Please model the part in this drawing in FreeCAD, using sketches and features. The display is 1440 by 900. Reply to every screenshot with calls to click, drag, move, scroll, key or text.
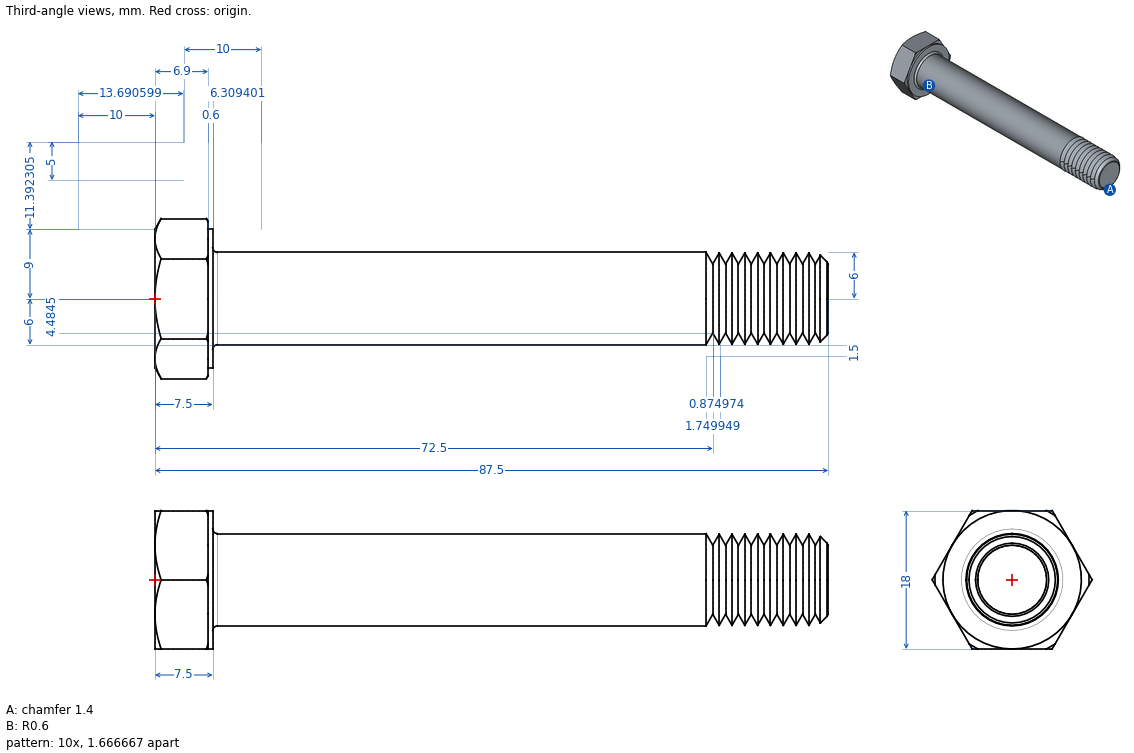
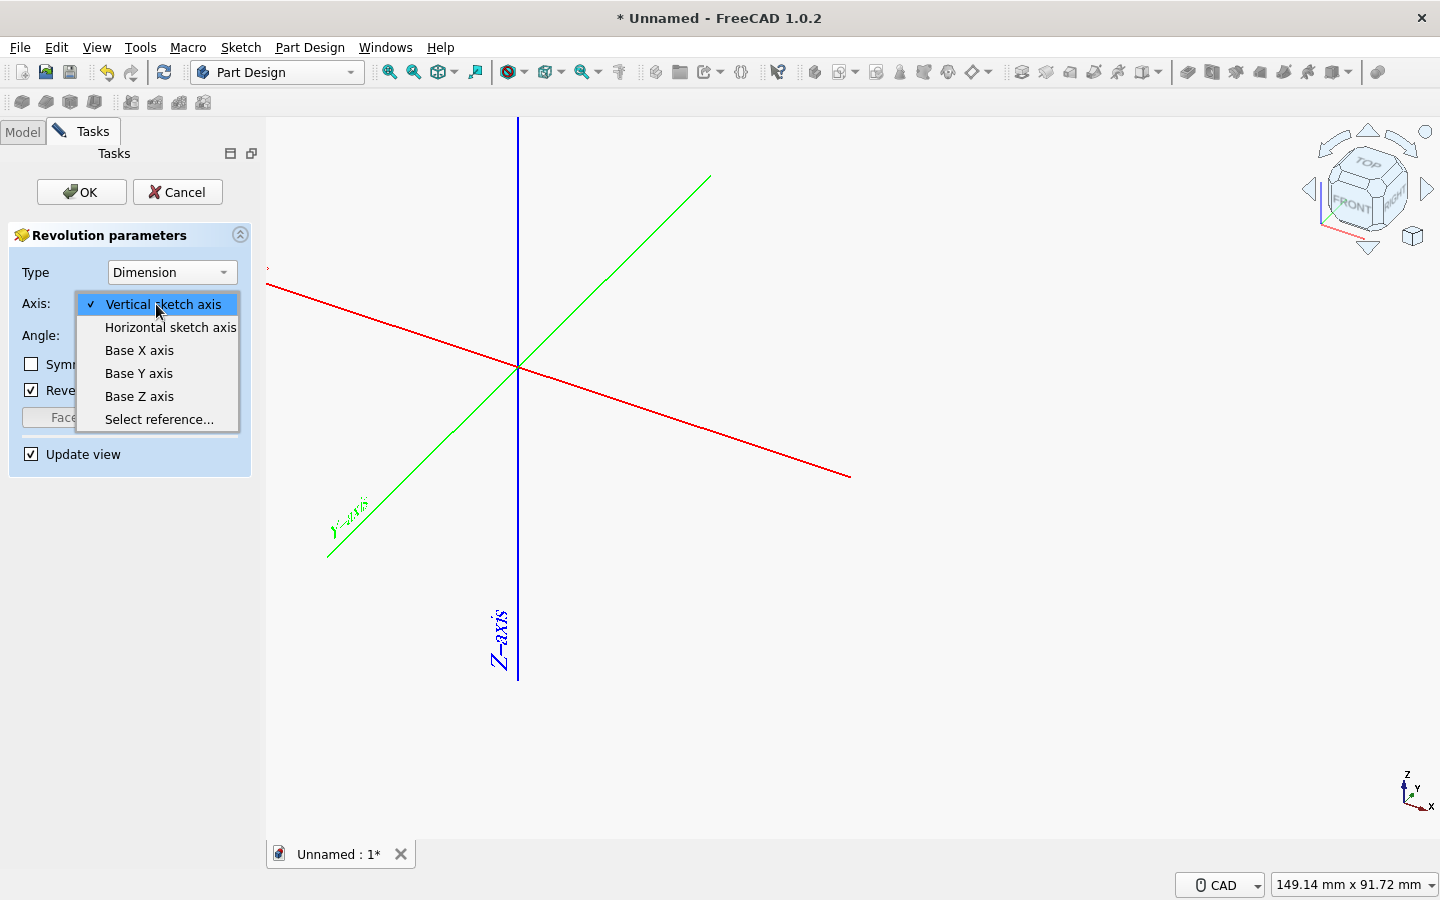
click(156, 328)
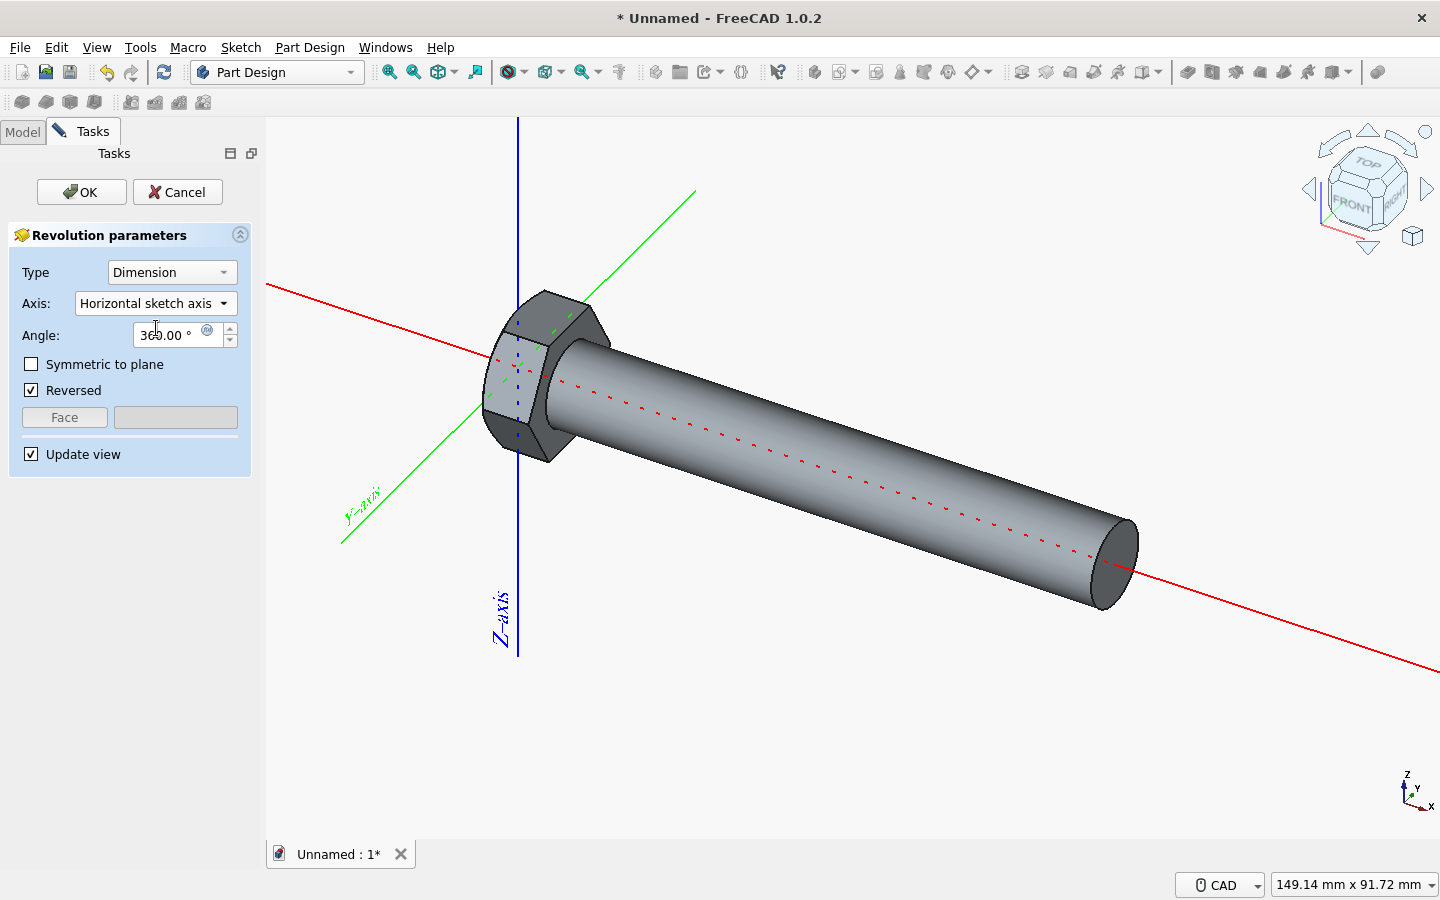
click(82, 192)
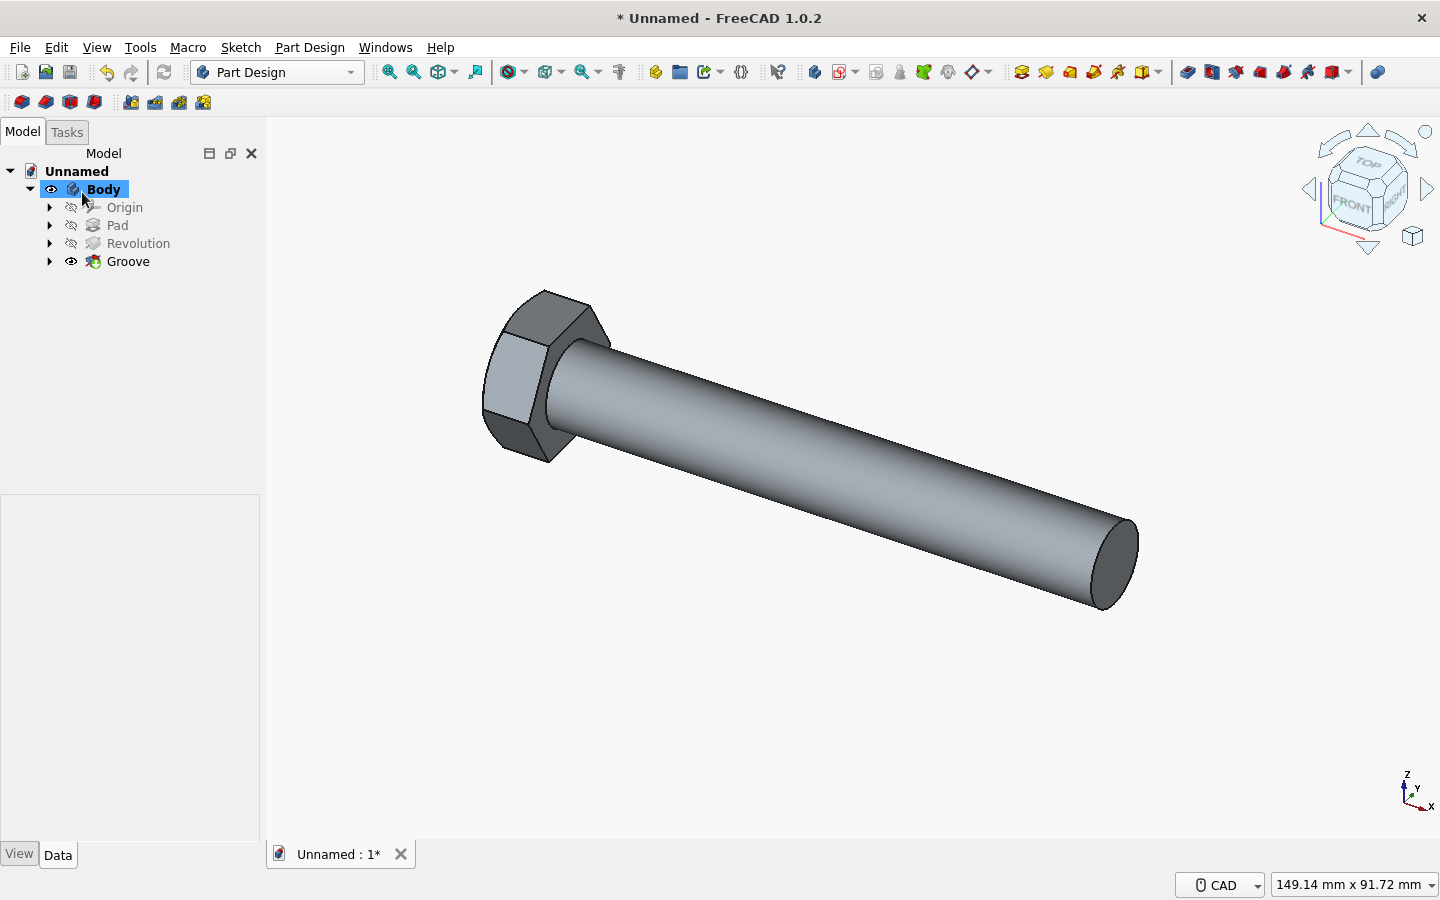
click(840, 72)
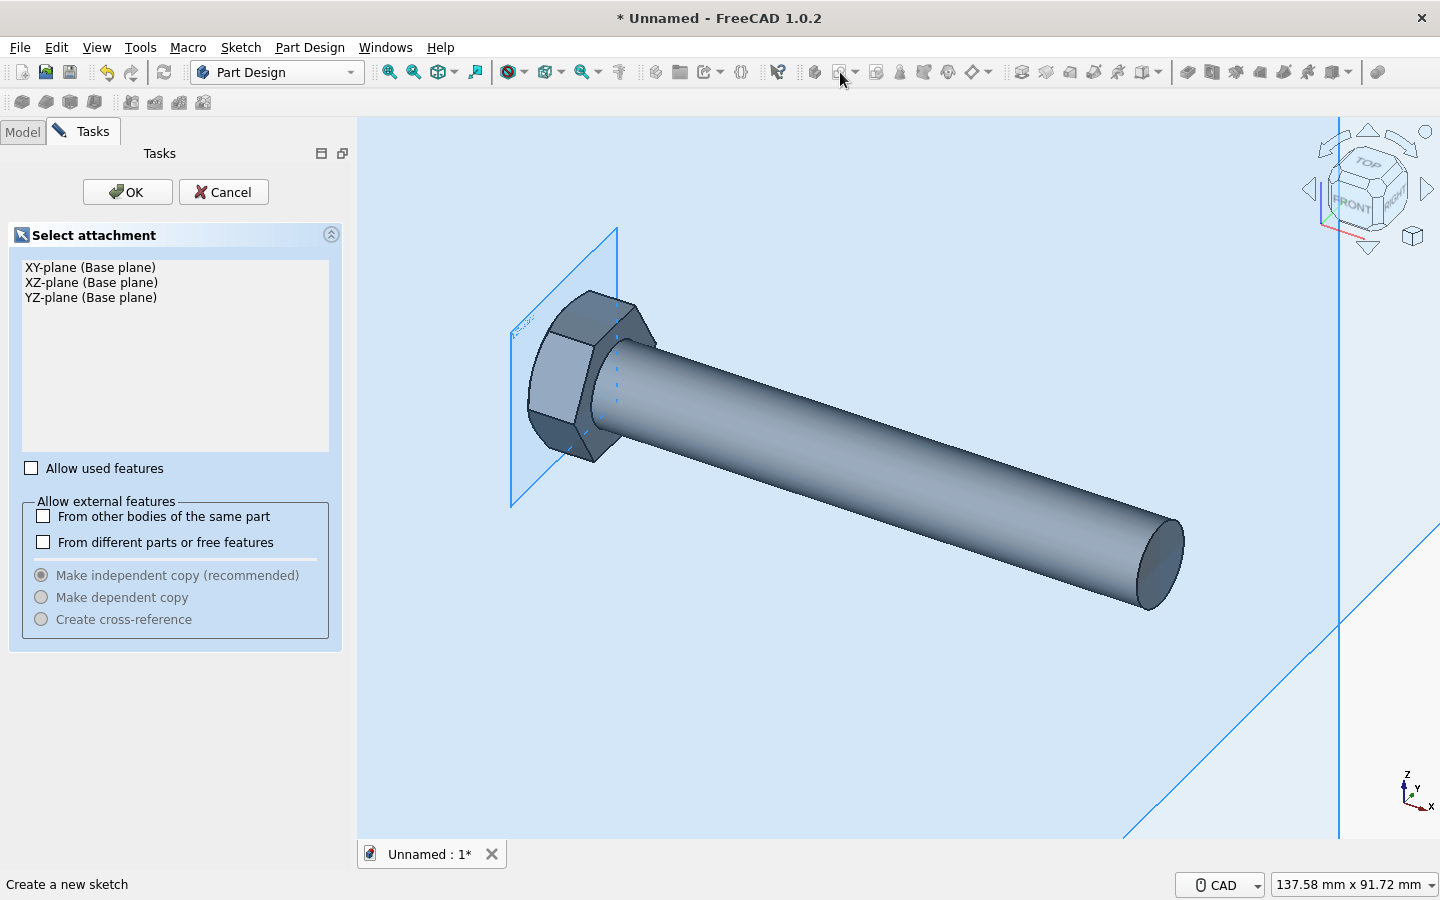
click(82, 268)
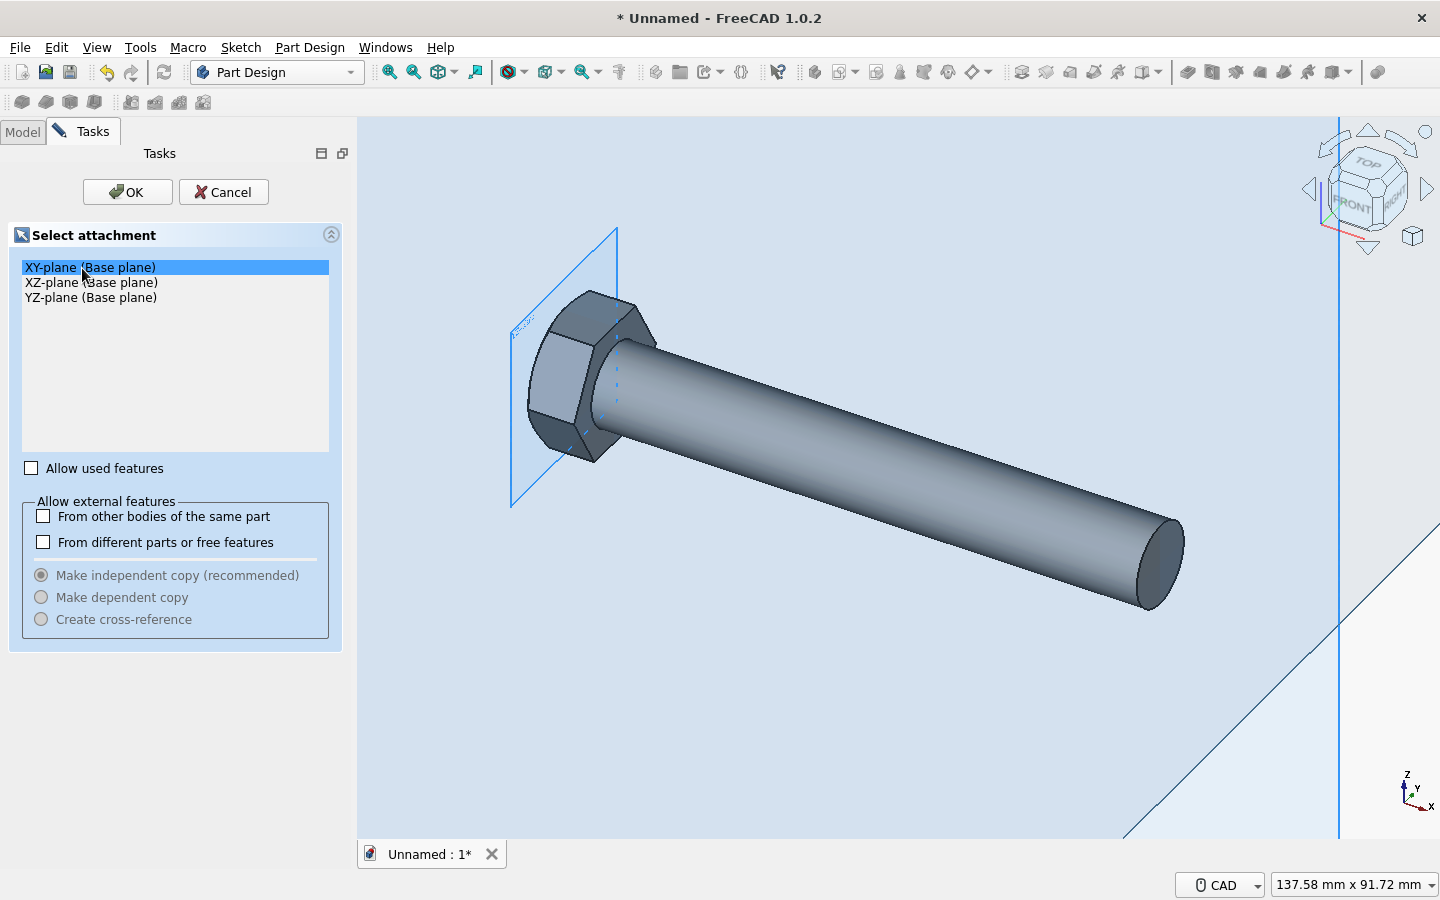
click(128, 192)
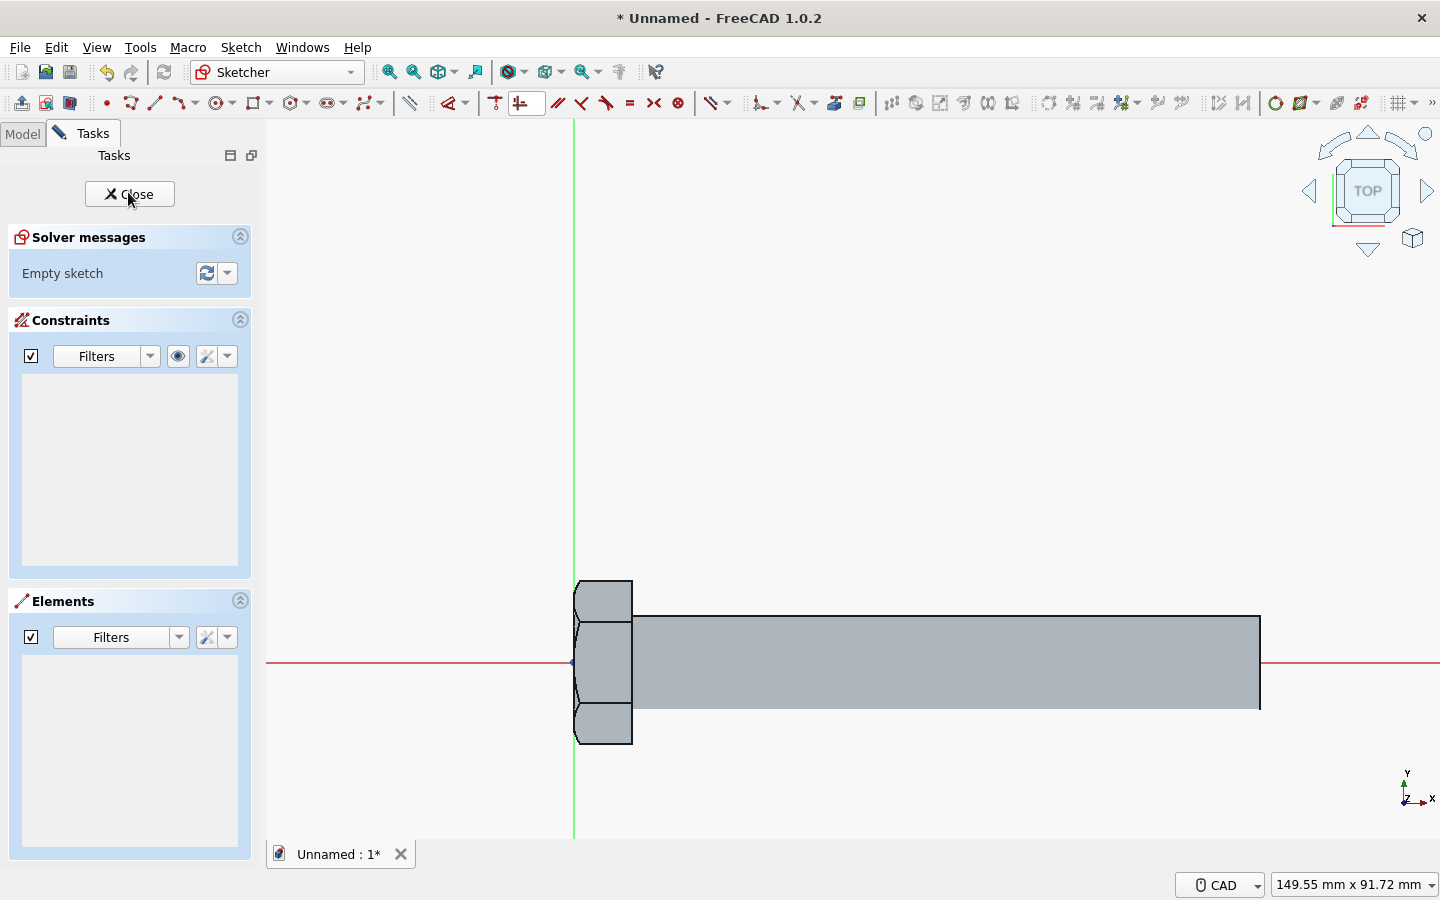
click(70, 104)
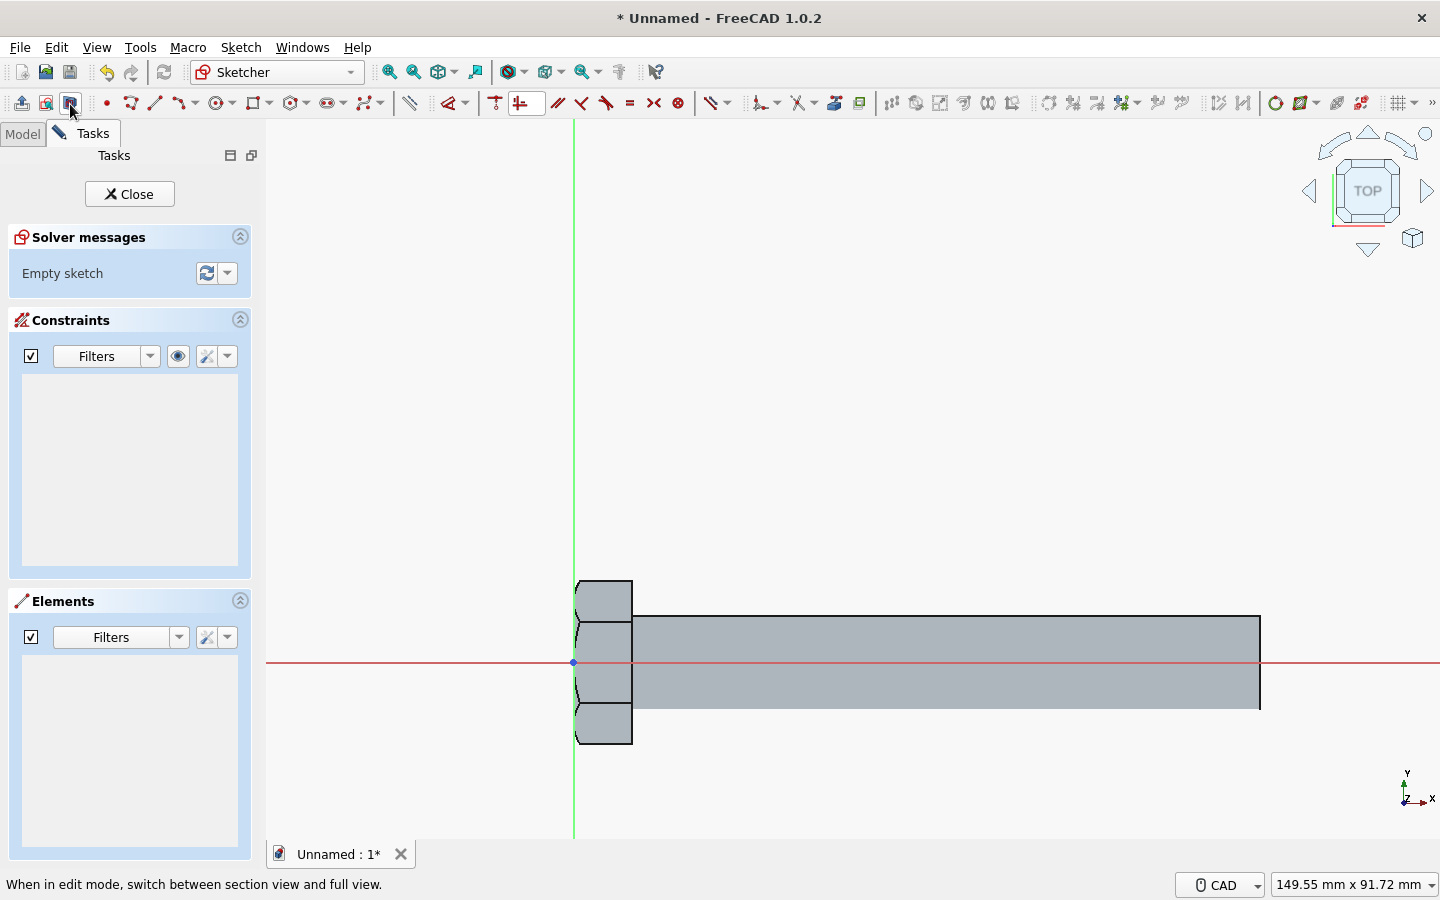
scroll(537, 643, up, 5)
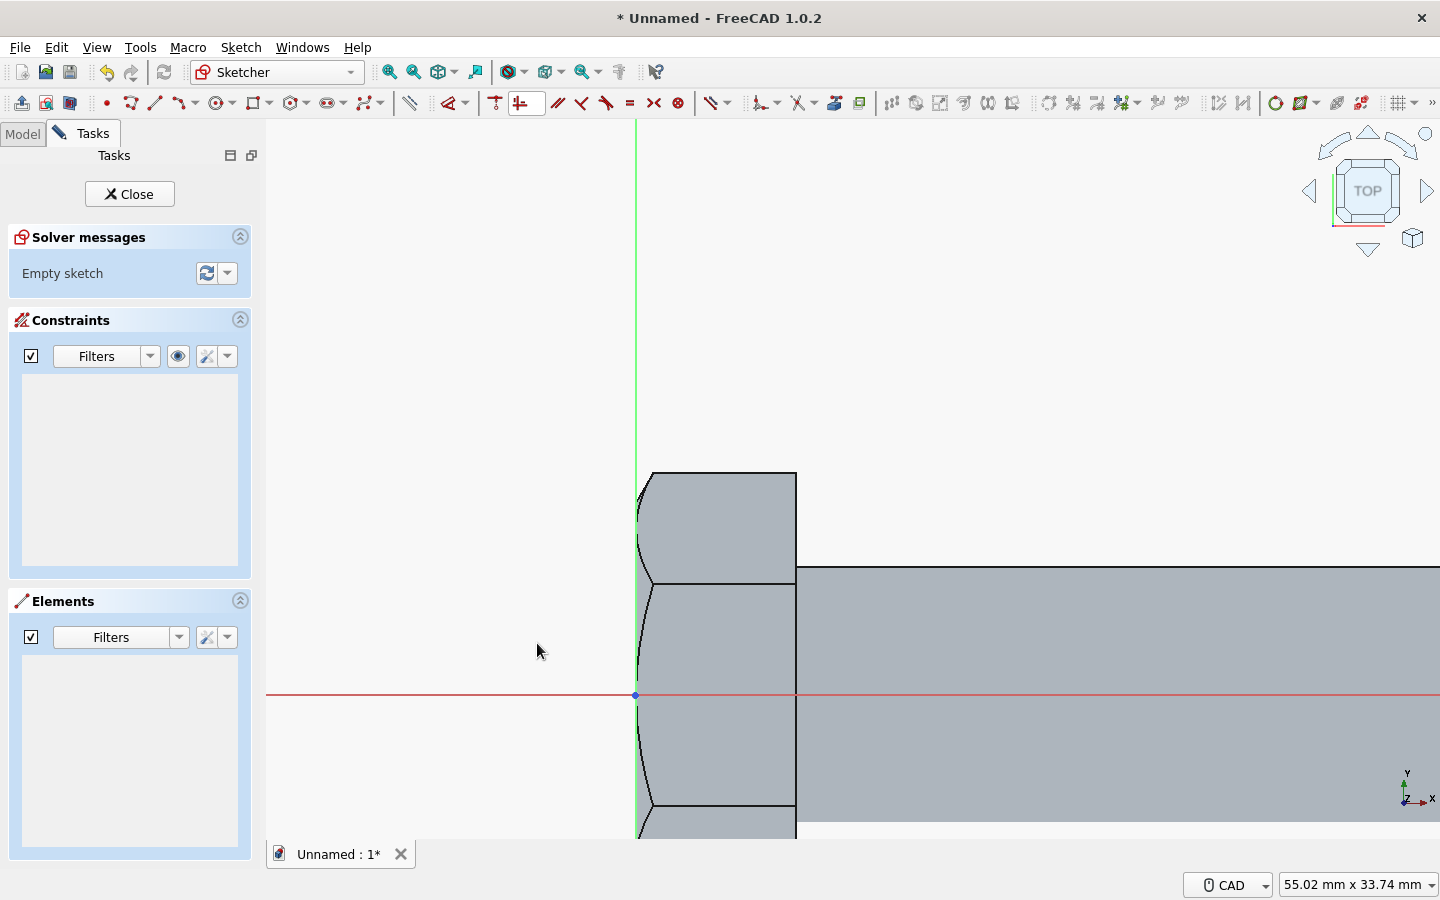
click(132, 104)